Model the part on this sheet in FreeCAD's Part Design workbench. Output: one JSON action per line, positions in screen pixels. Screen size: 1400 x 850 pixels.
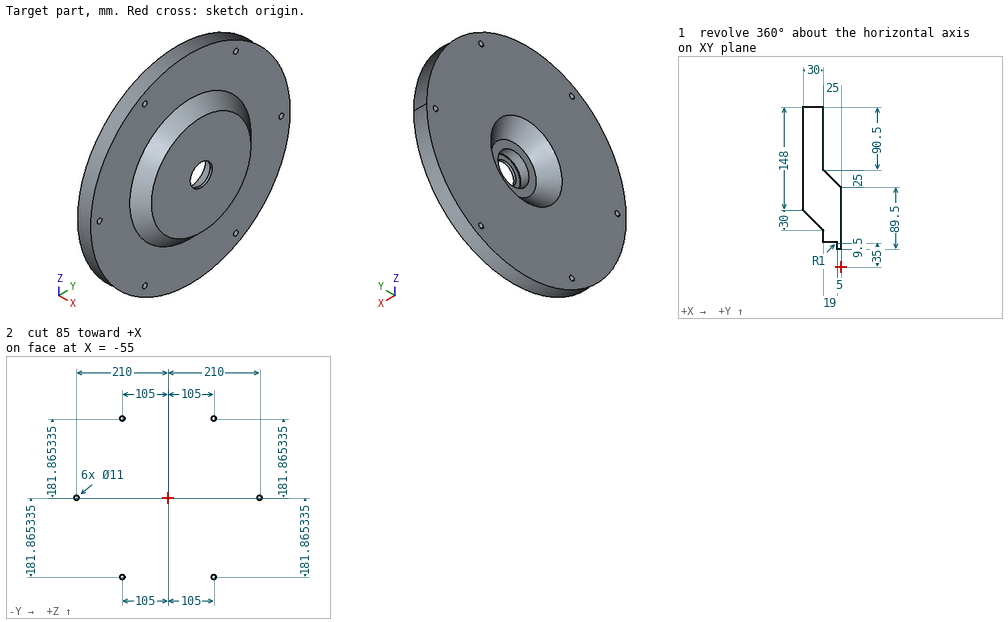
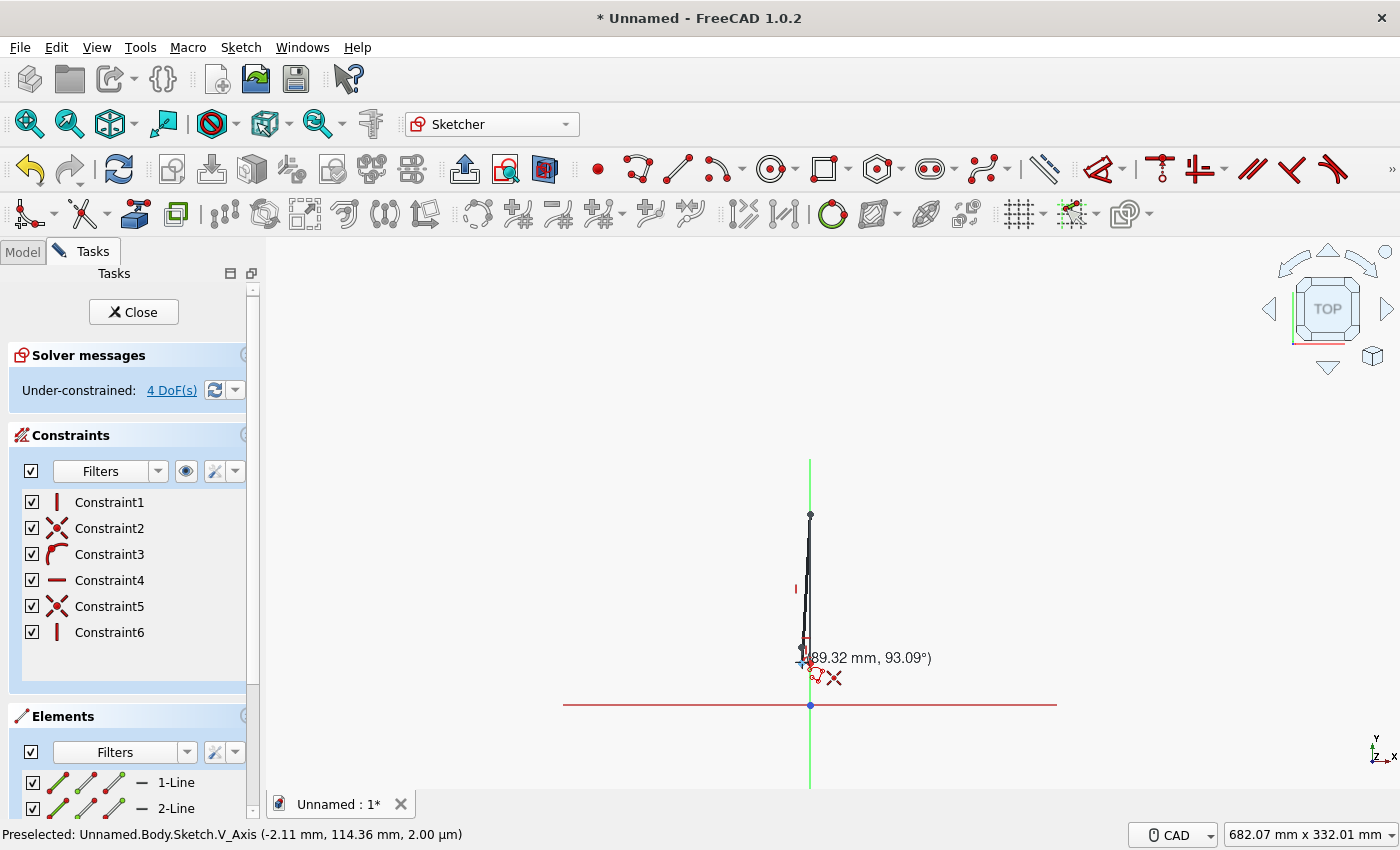
{"action": "left_click", "coordinate": [769, 472]}
{"action": "left_click", "coordinate": [769, 322]}
{"action": "left_click", "coordinate": [719, 322]}
{"action": "left_click", "coordinate": [719, 568]}
{"action": "left_click", "coordinate": [769, 618]}
{"action": "left_click", "coordinate": [769, 645]}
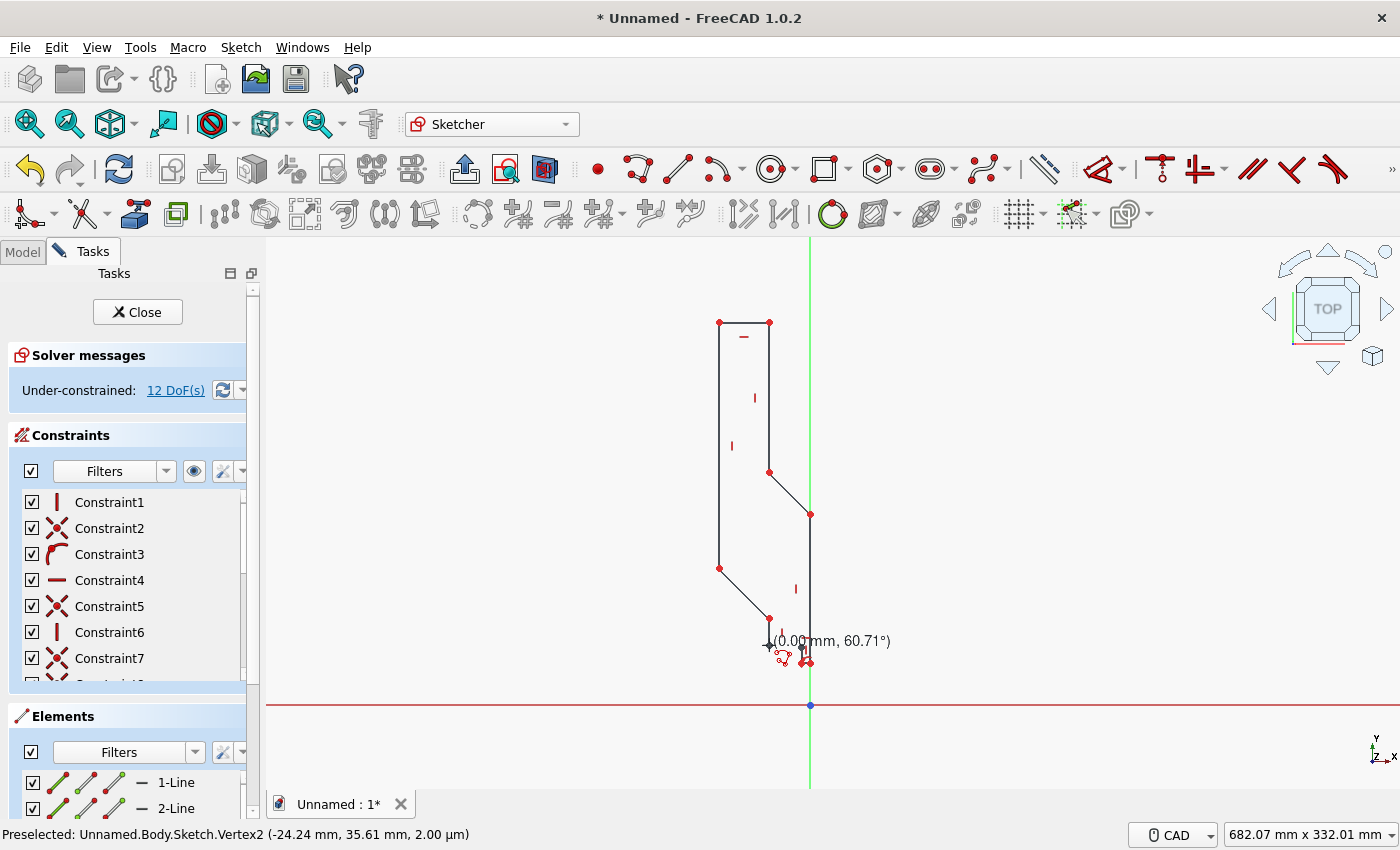
{"action": "scroll", "coordinate": [800, 645], "scroll_direction": "up", "scroll_amount": 10}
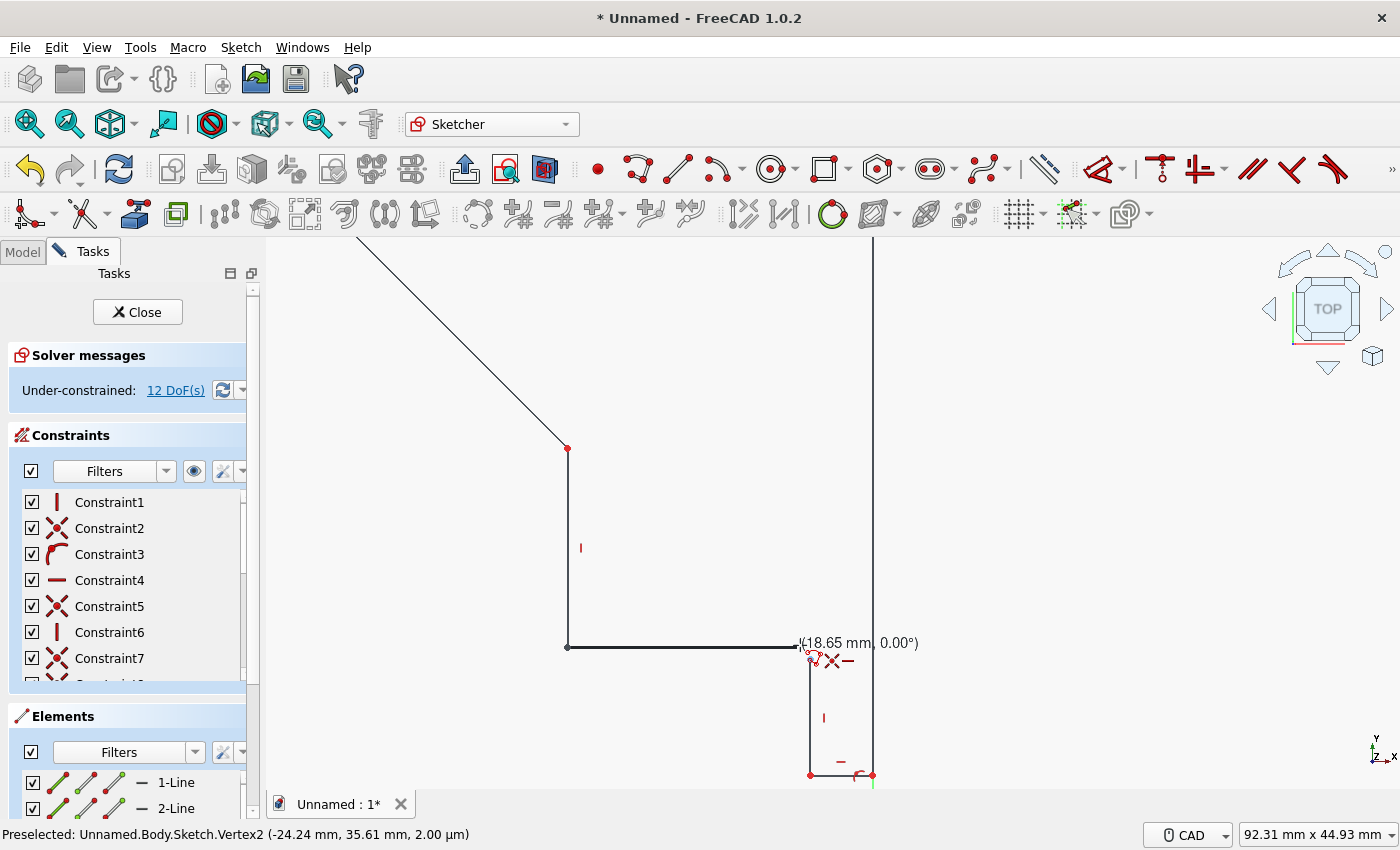
{"action": "left_click", "coordinate": [799, 640]}
{"action": "right_click", "coordinate": [799, 640]}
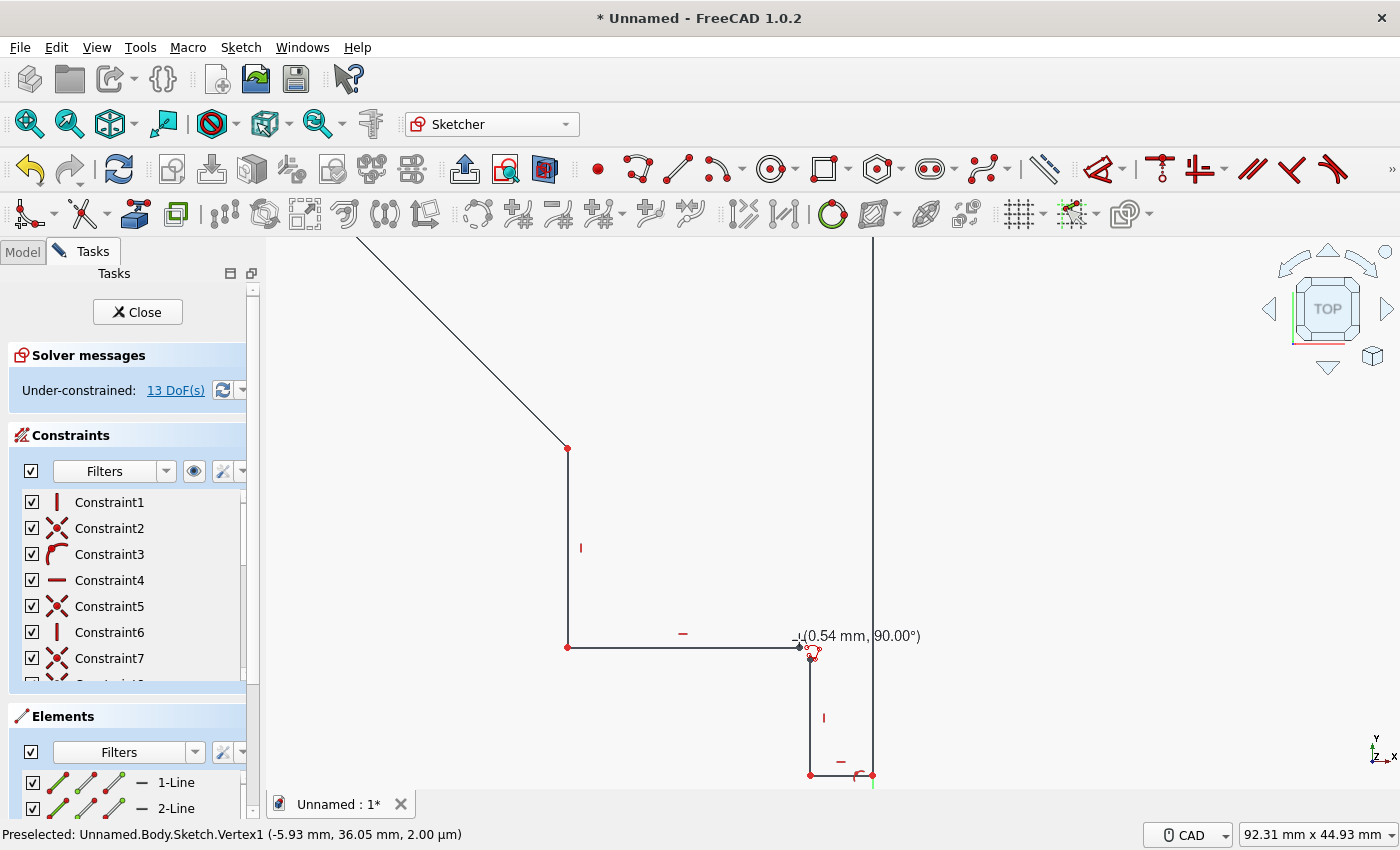
{"action": "left_click", "coordinate": [744, 170]}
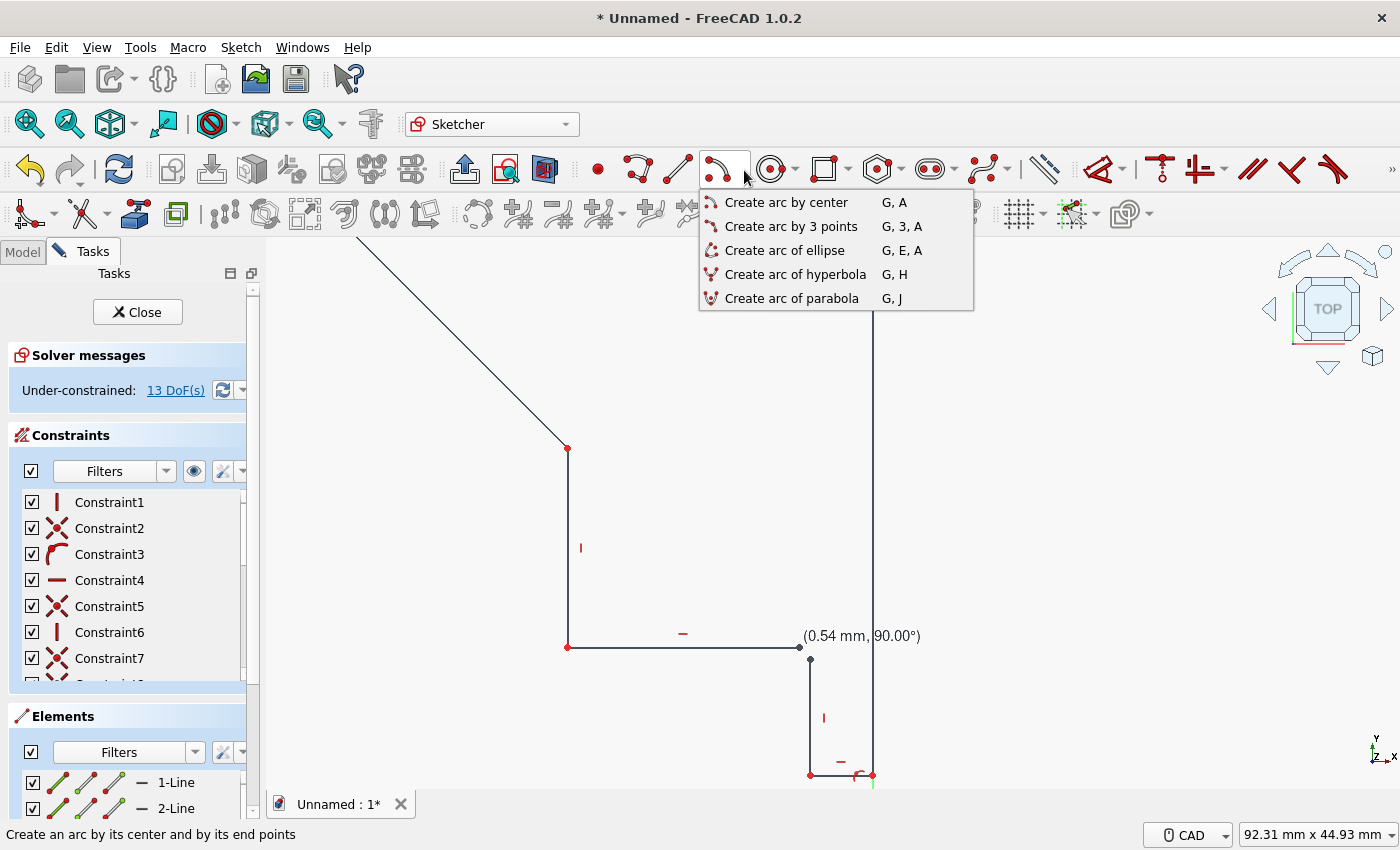
{"action": "left_click", "coordinate": [836, 226]}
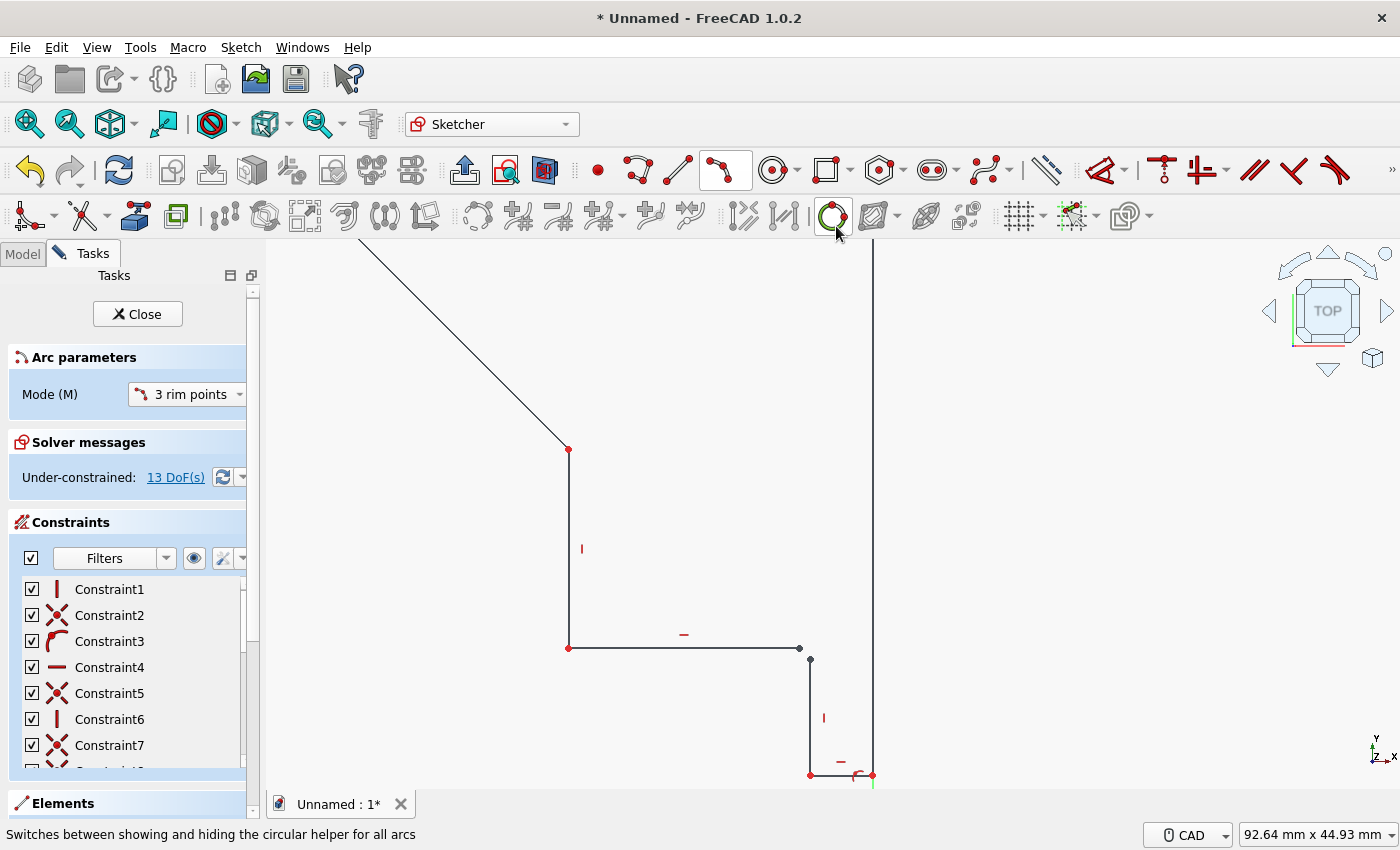
{"action": "left_click", "coordinate": [799, 648]}
{"action": "left_click", "coordinate": [810, 660]}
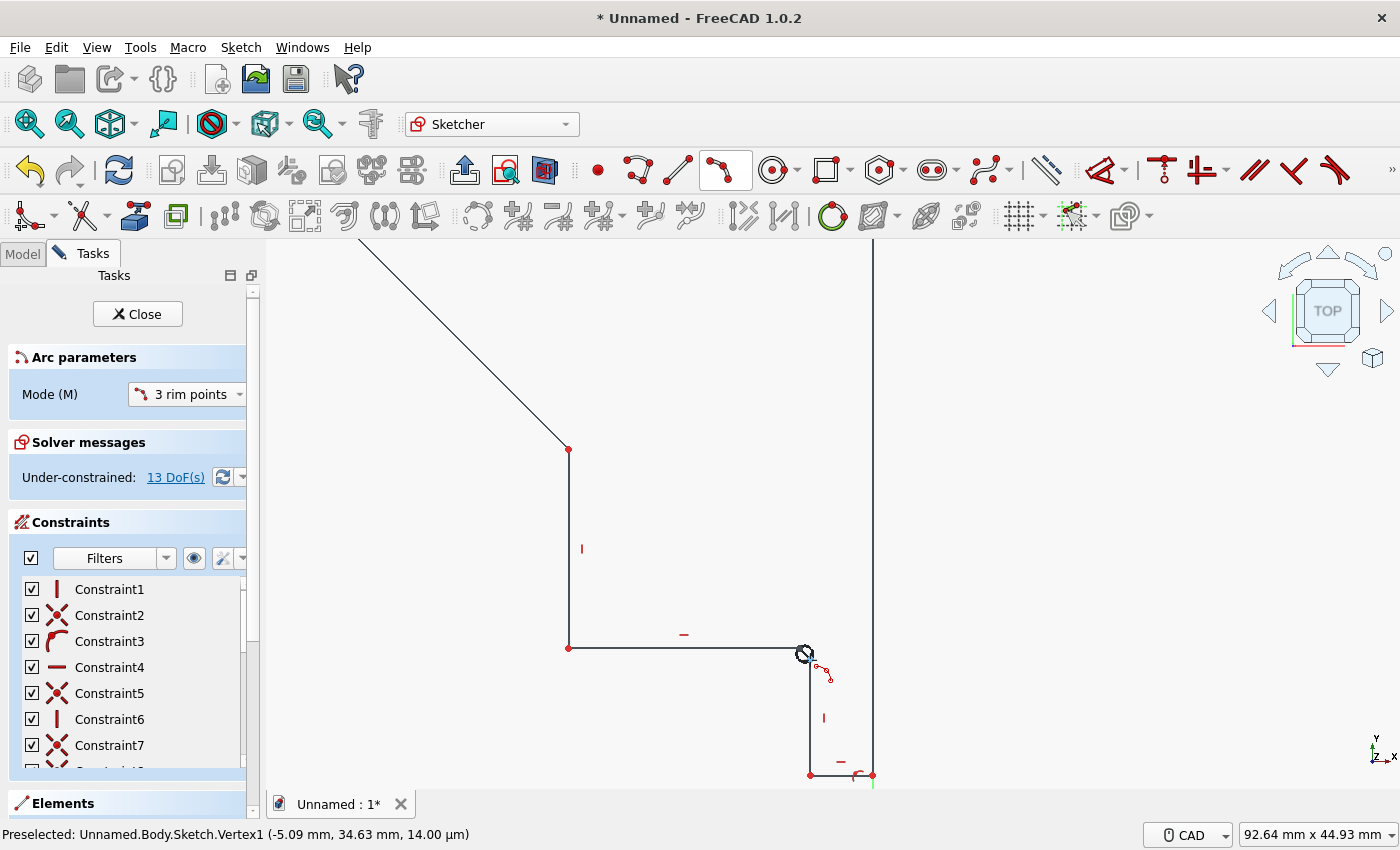
{"action": "scroll", "coordinate": [808, 647], "scroll_direction": "up", "scroll_amount": 8}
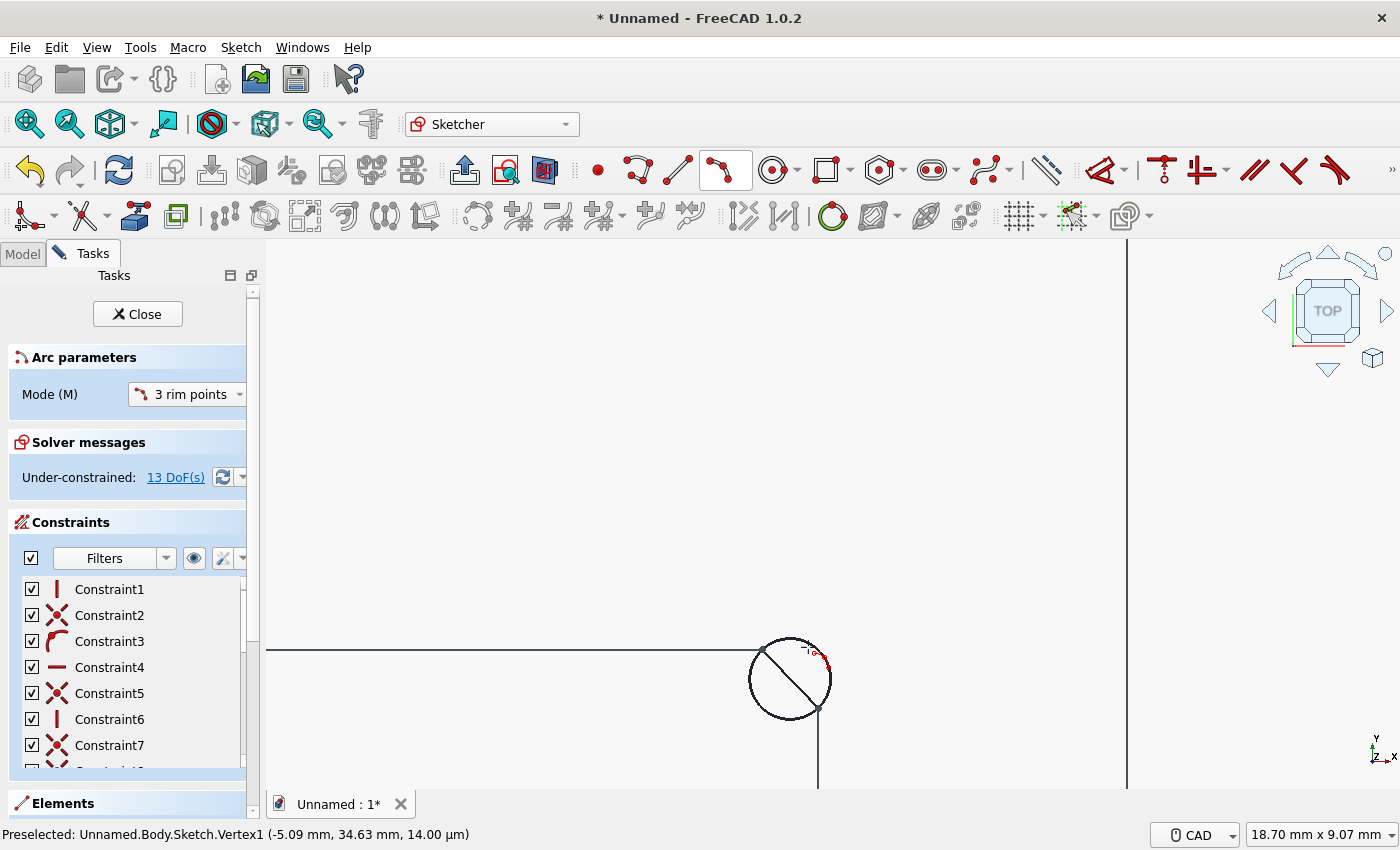
{"action": "left_click", "coordinate": [806, 643]}
{"action": "key", "text": "Escape"}